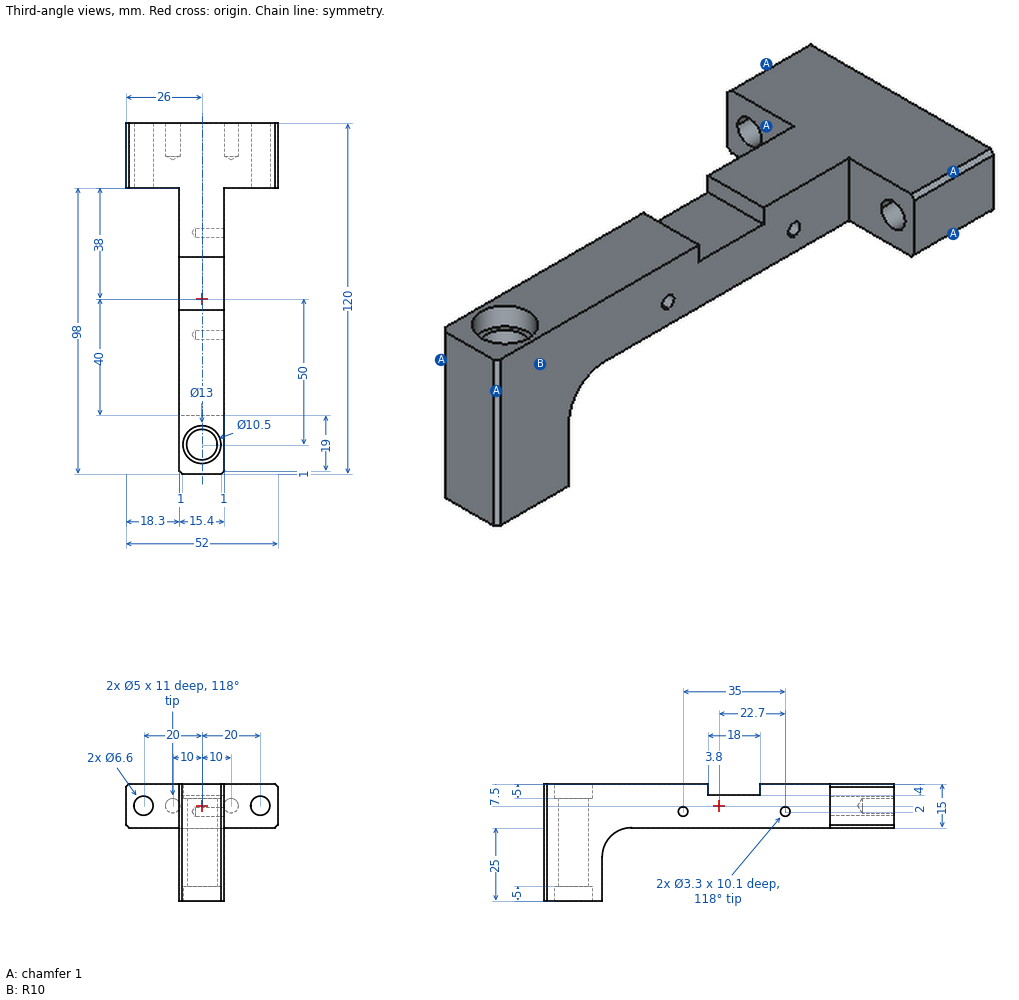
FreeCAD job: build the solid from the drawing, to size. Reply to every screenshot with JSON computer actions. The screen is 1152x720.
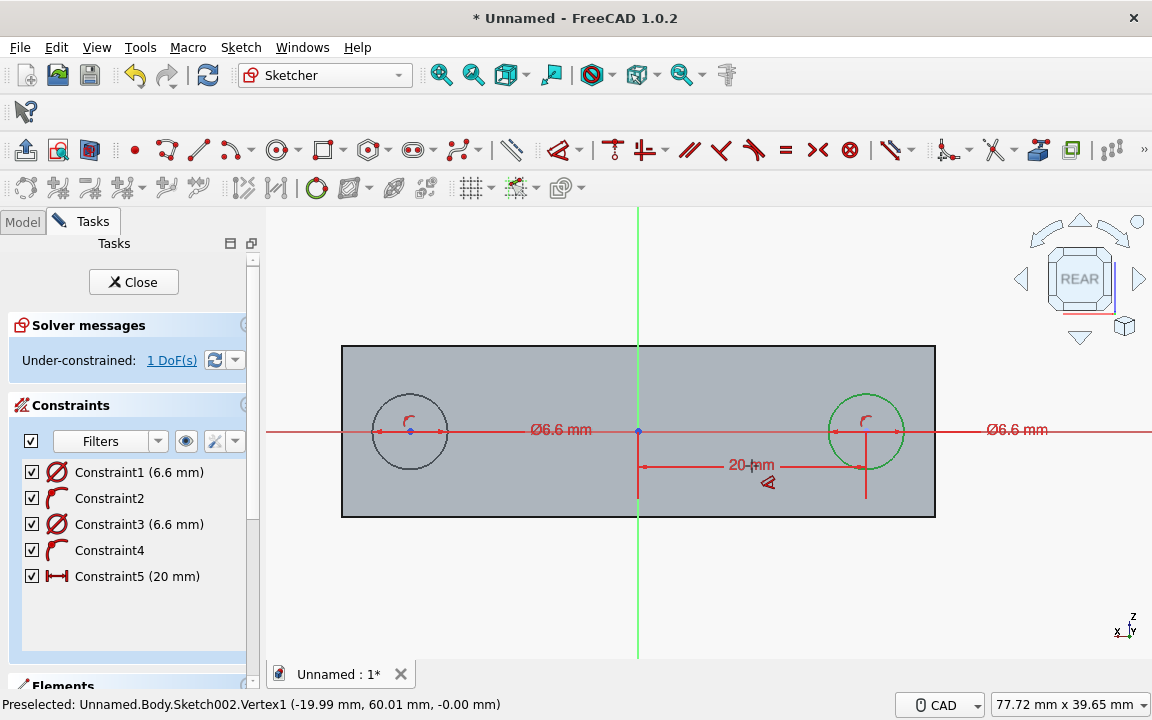
{"action": "left_click", "coordinate": [410, 432]}
{"action": "left_click", "coordinate": [524, 466]}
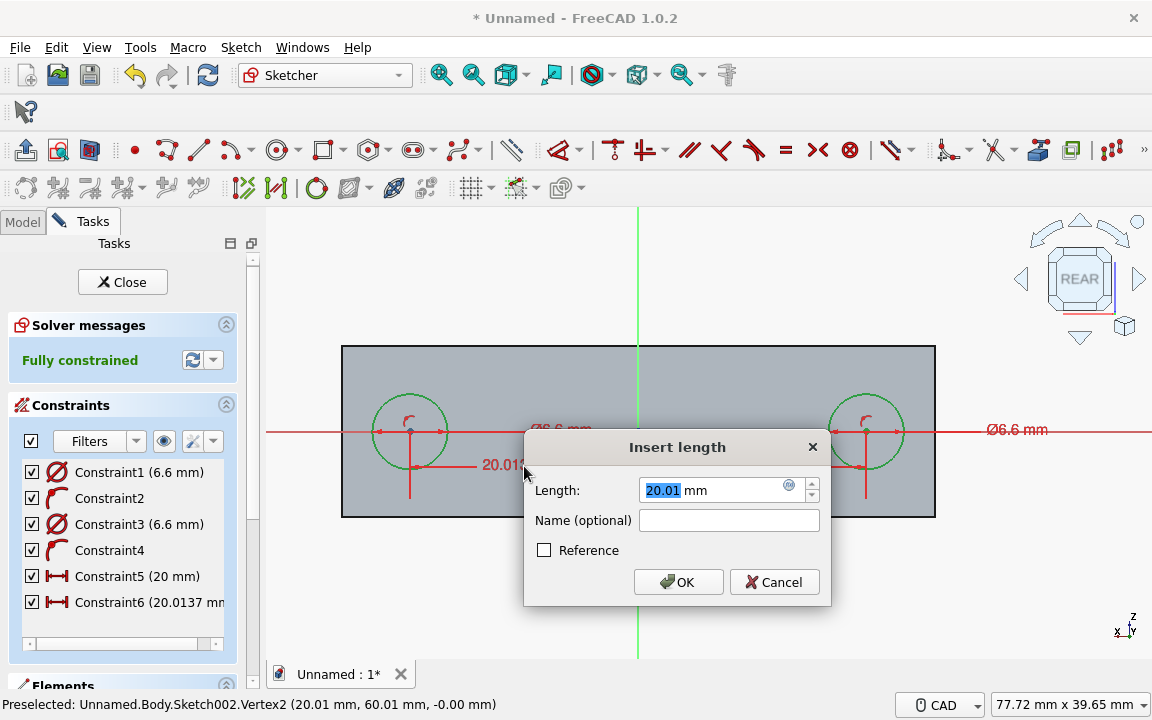
{"action": "type", "text": "20"}
{"action": "key", "text": "Return"}
{"action": "key", "text": "Escape"}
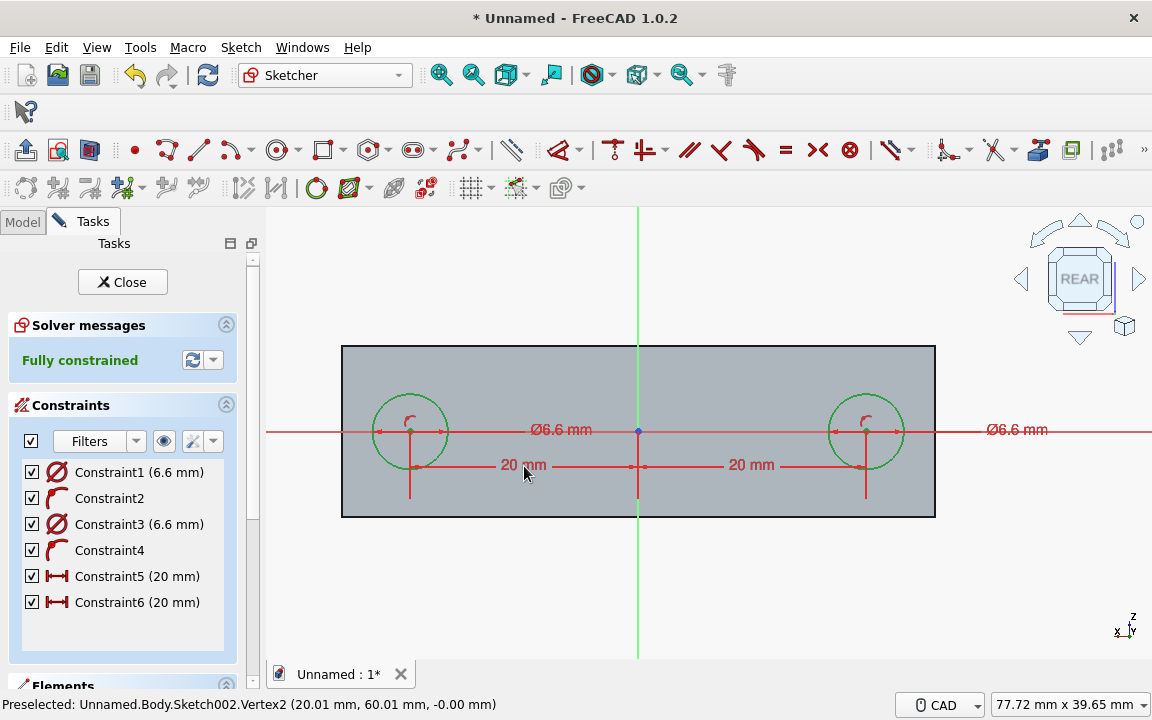
{"action": "left_click", "coordinate": [123, 282]}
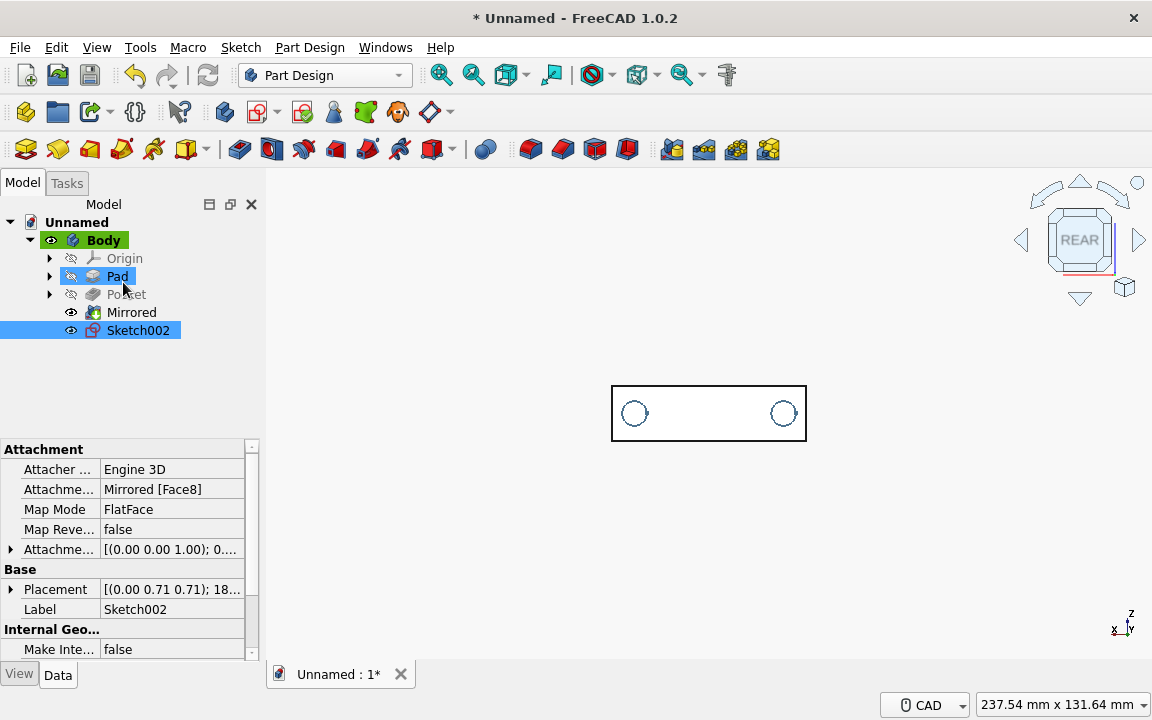
{"action": "left_click", "coordinate": [240, 150]}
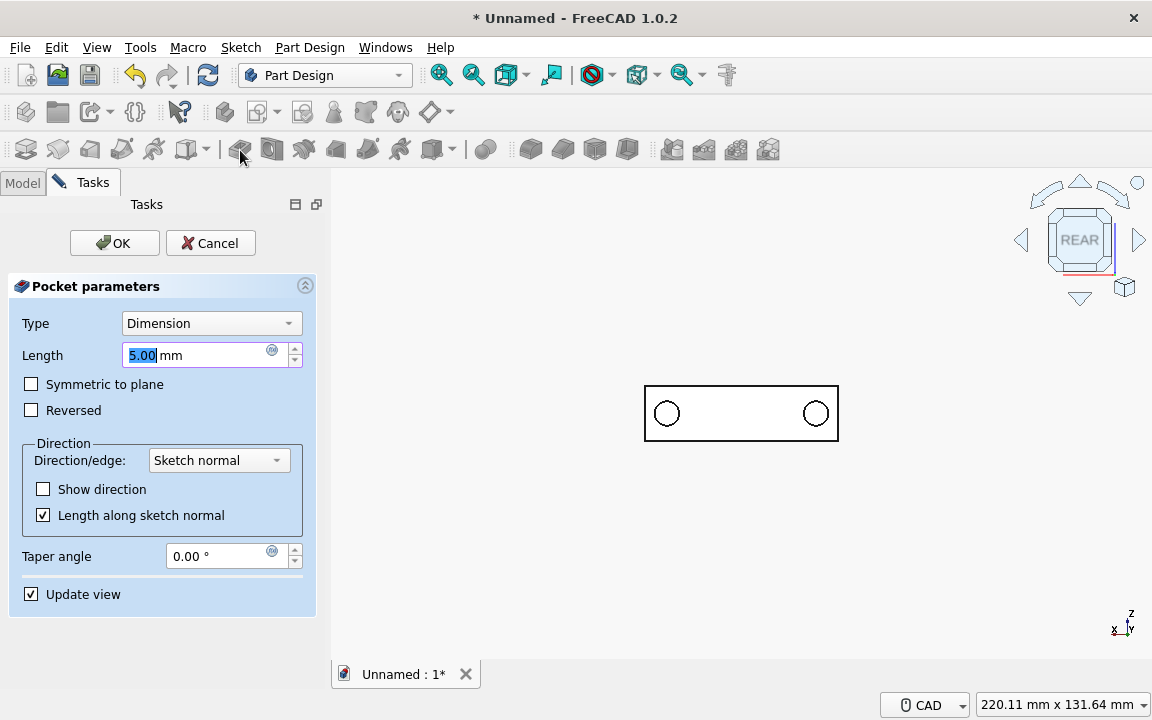
{"action": "left_click", "coordinate": [212, 324]}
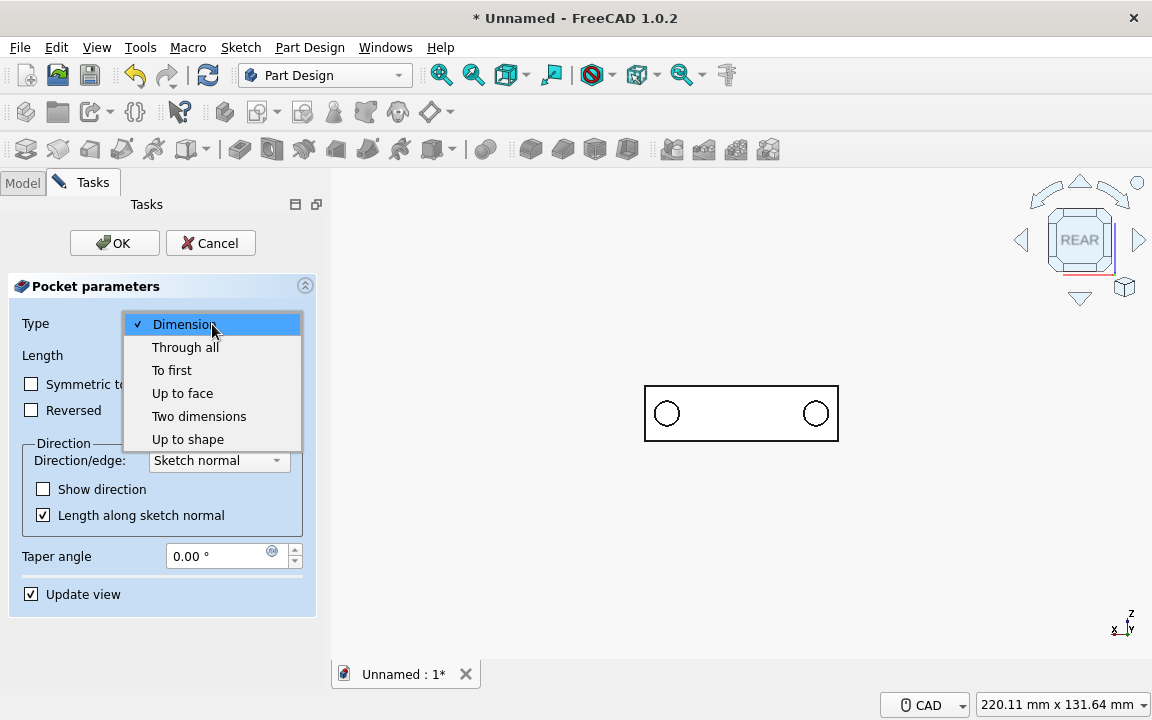
{"action": "left_click", "coordinate": [212, 348]}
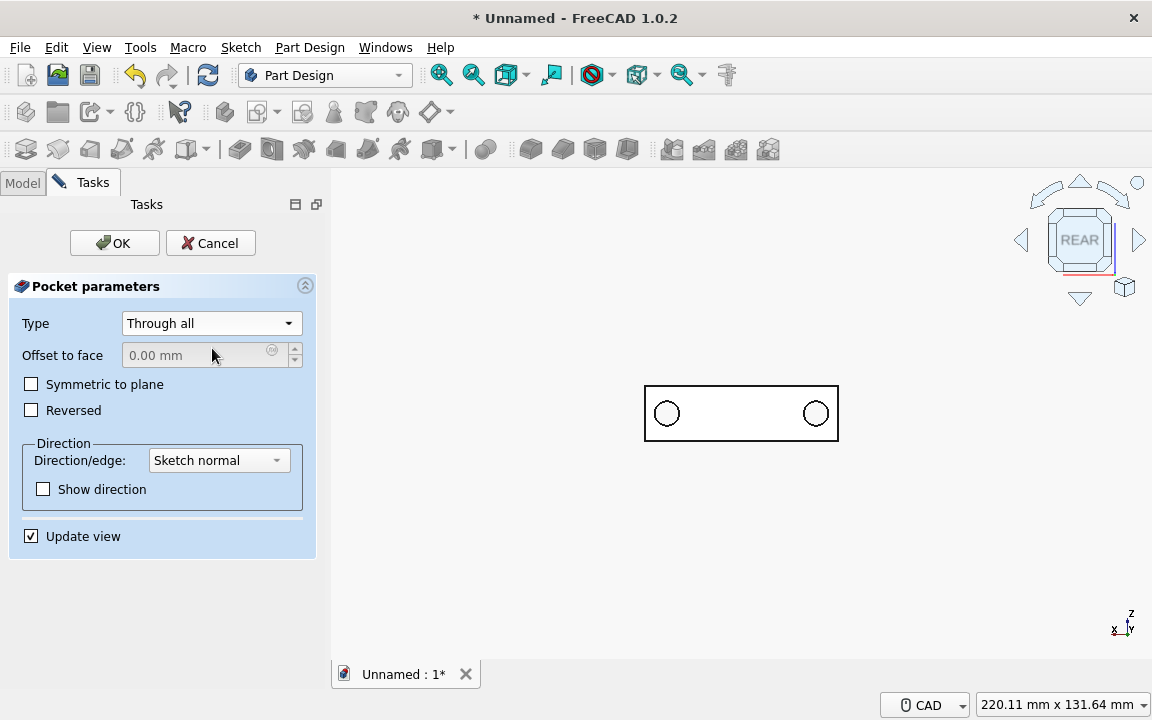
{"action": "left_click", "coordinate": [115, 243]}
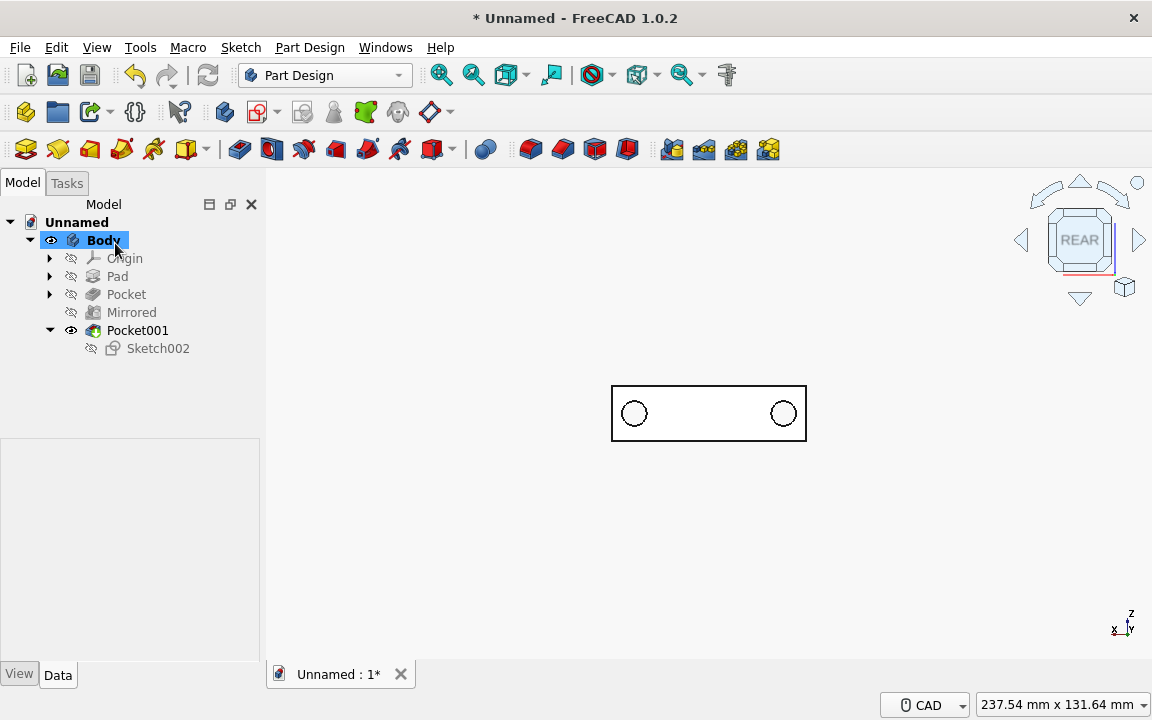
{"action": "left_click", "coordinate": [442, 76]}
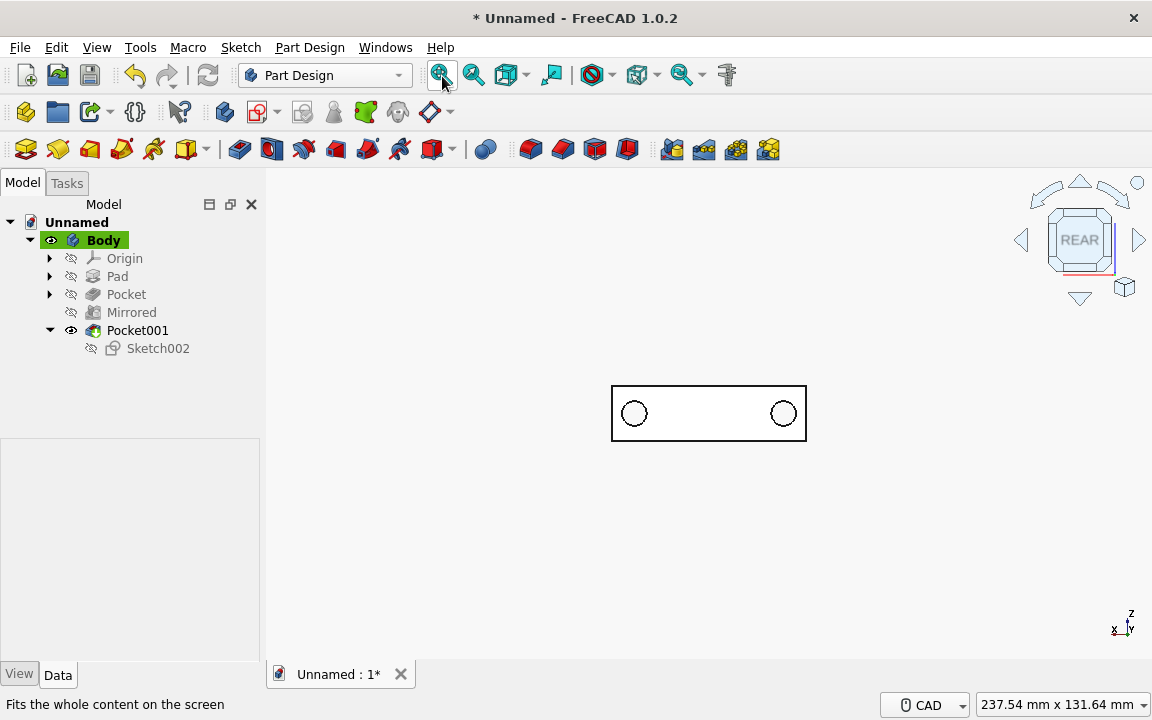
{"action": "key", "text": "0"}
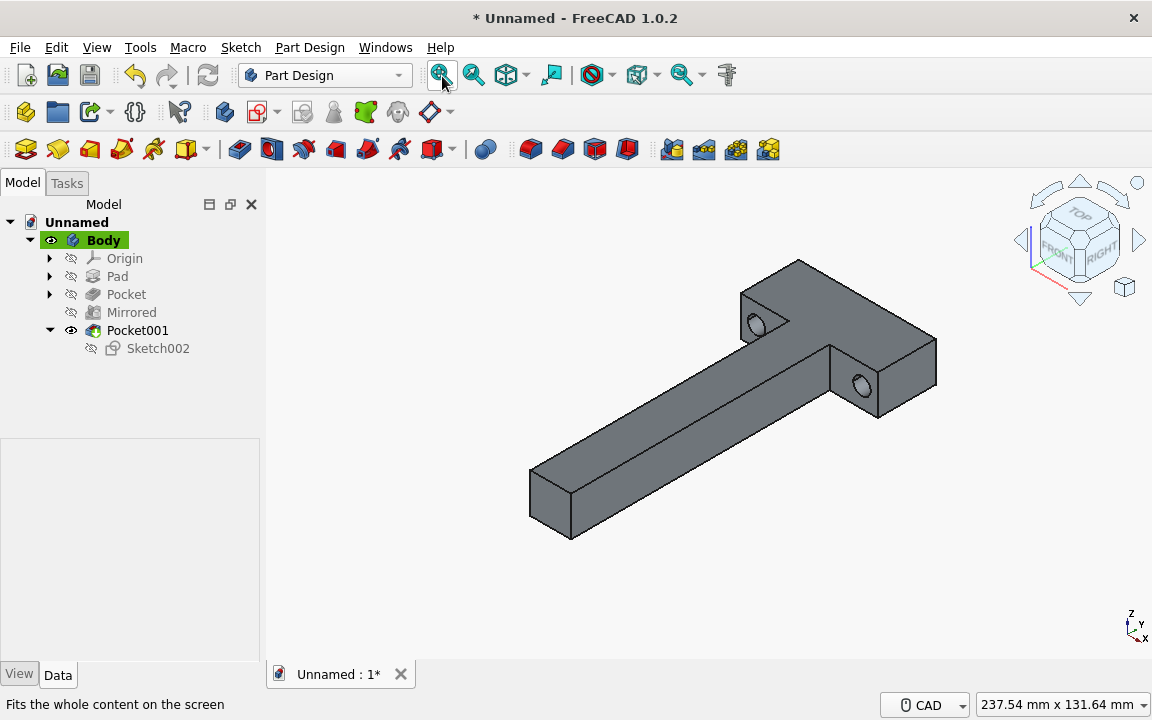
{"action": "left_click", "coordinate": [907, 355]}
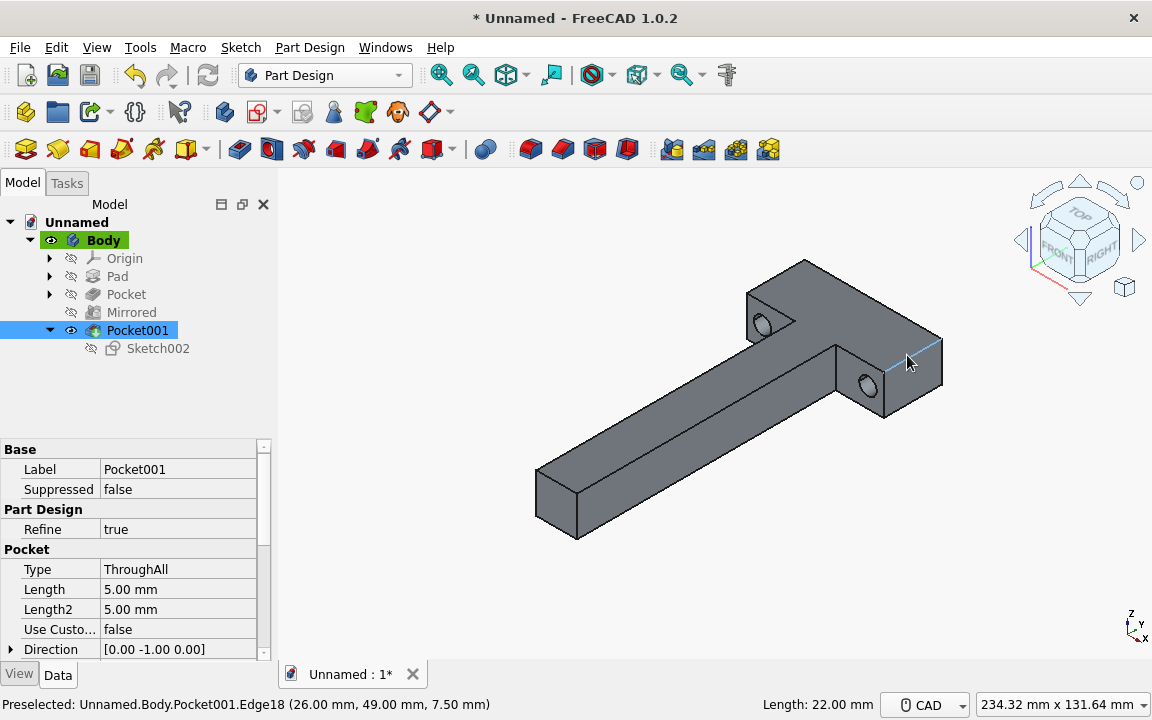
{"action": "left_click", "coordinate": [577, 516], "text": "ctrl"}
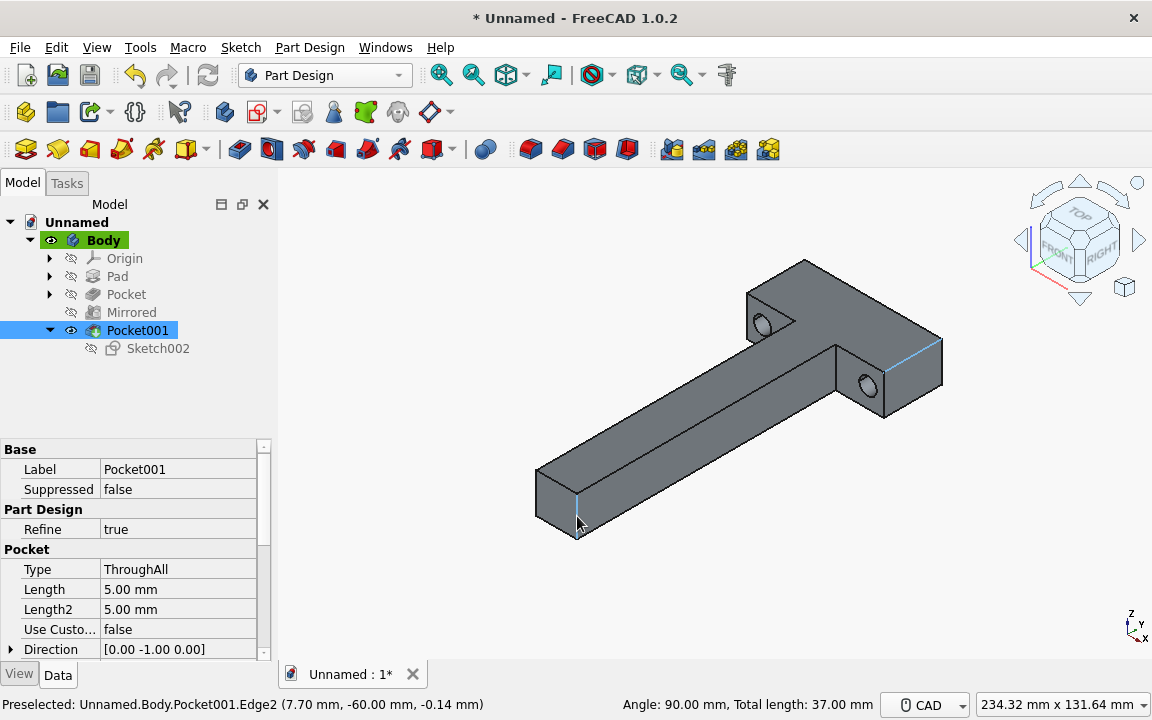
{"action": "key", "text": "2"}